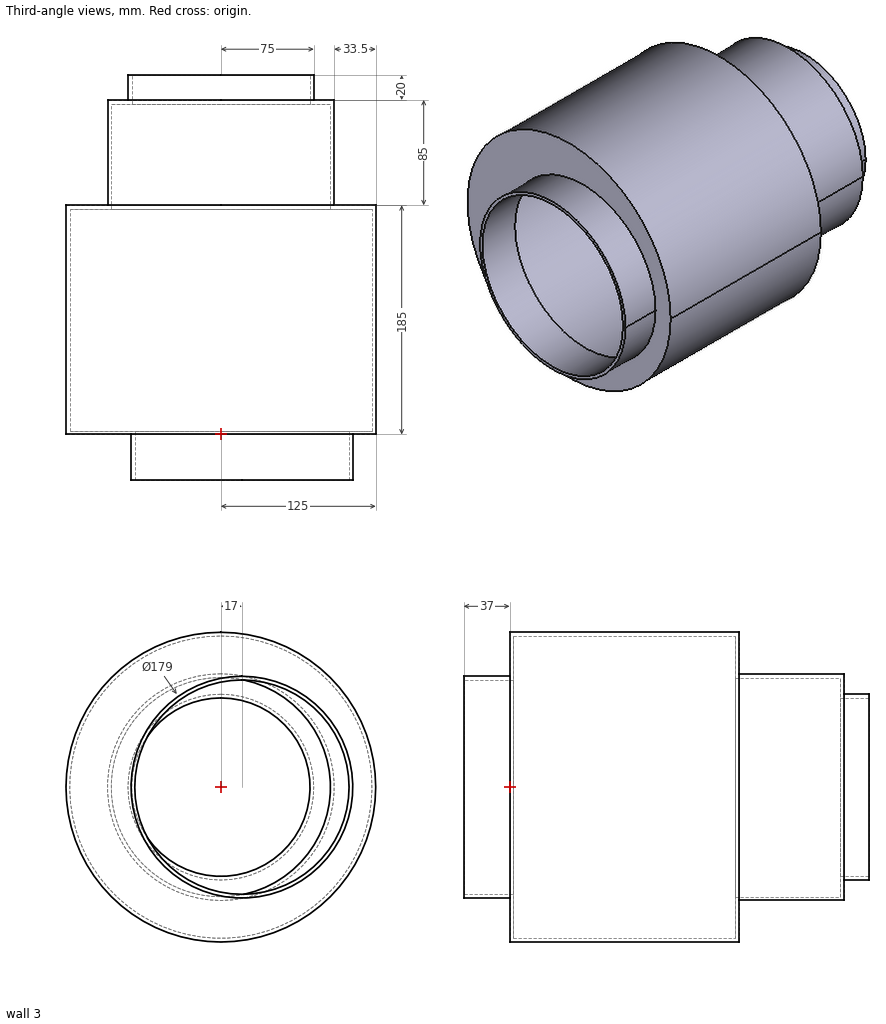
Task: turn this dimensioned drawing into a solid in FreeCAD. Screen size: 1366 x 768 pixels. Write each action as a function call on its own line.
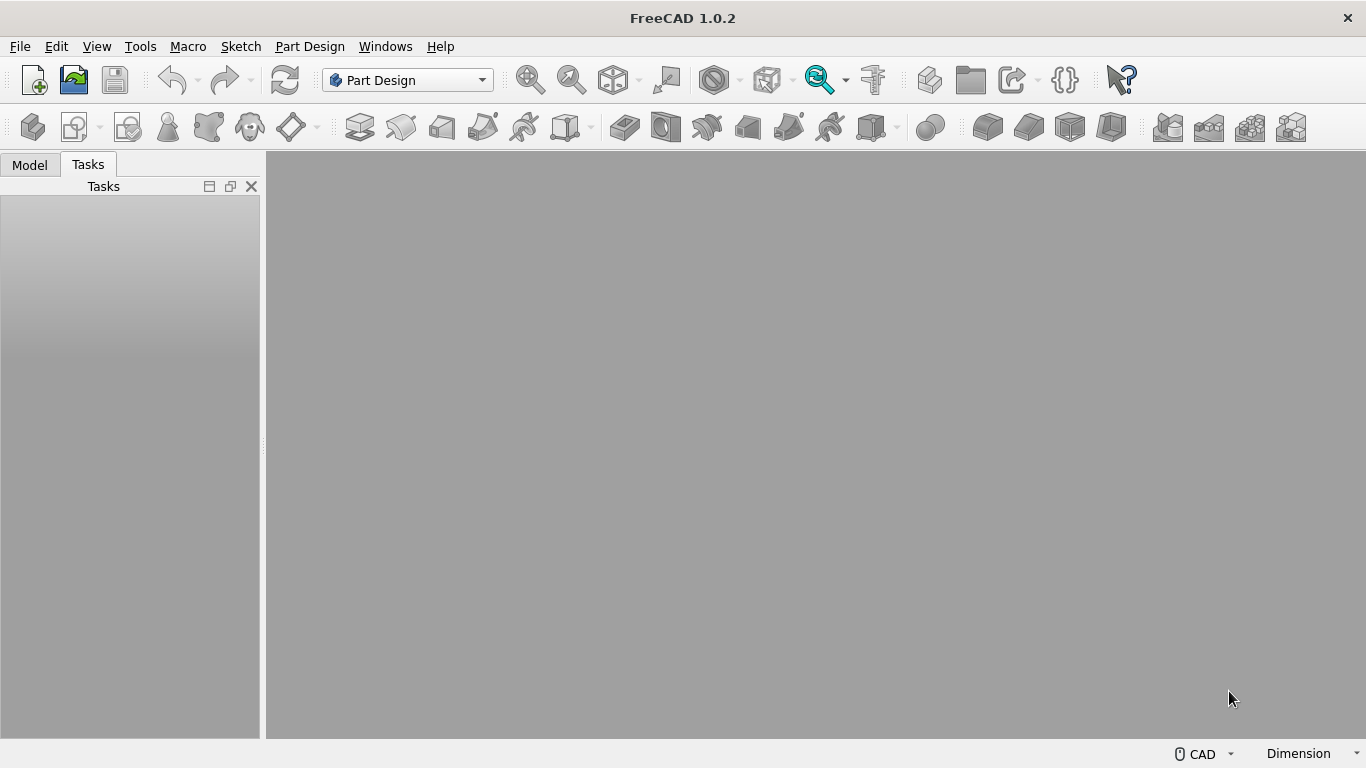
click(33, 80)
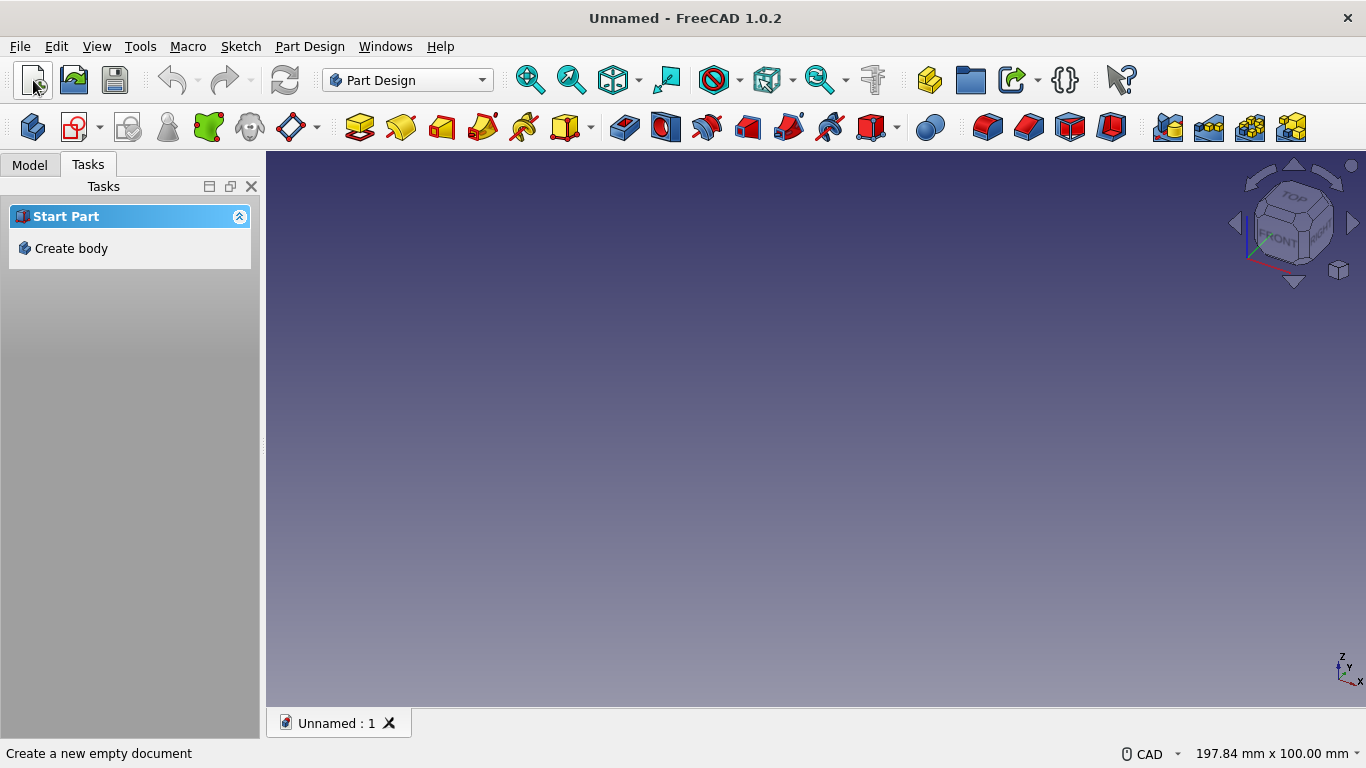
click(74, 128)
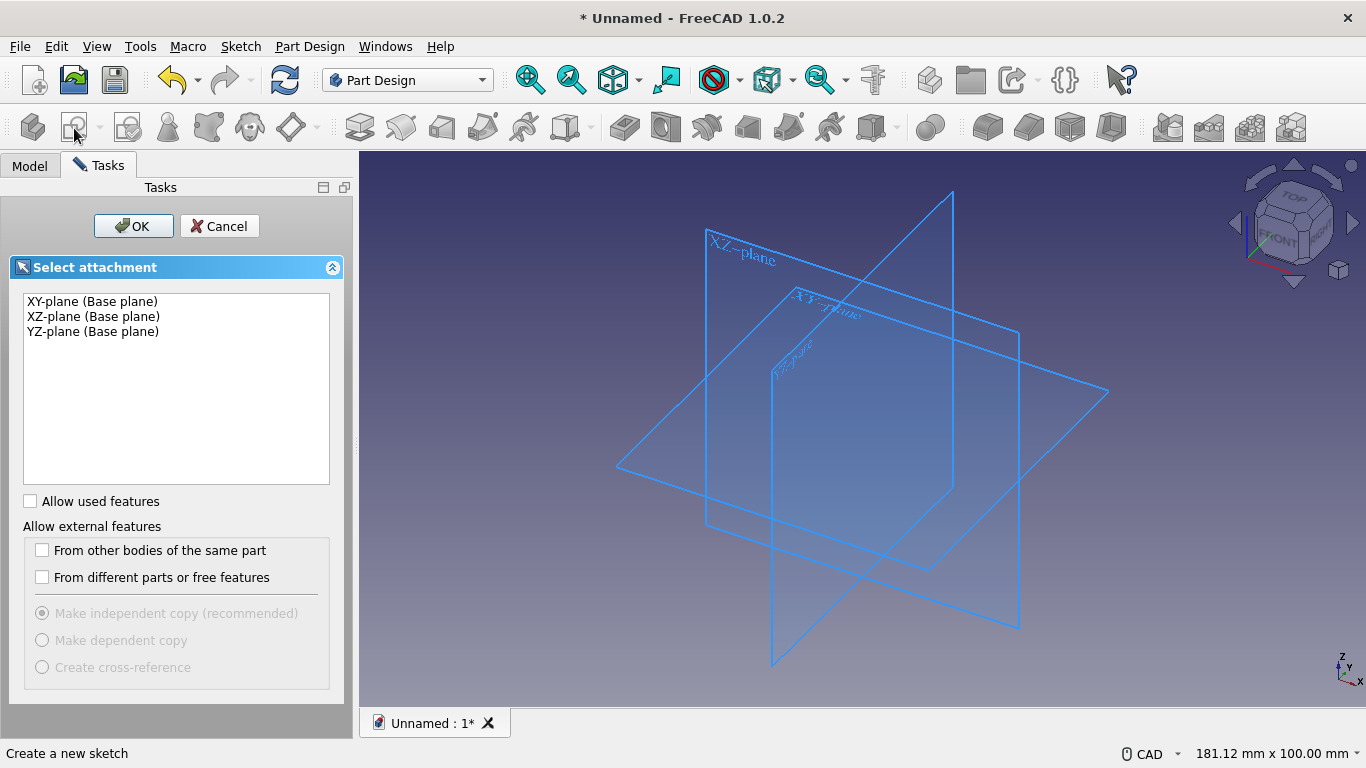
click(84, 302)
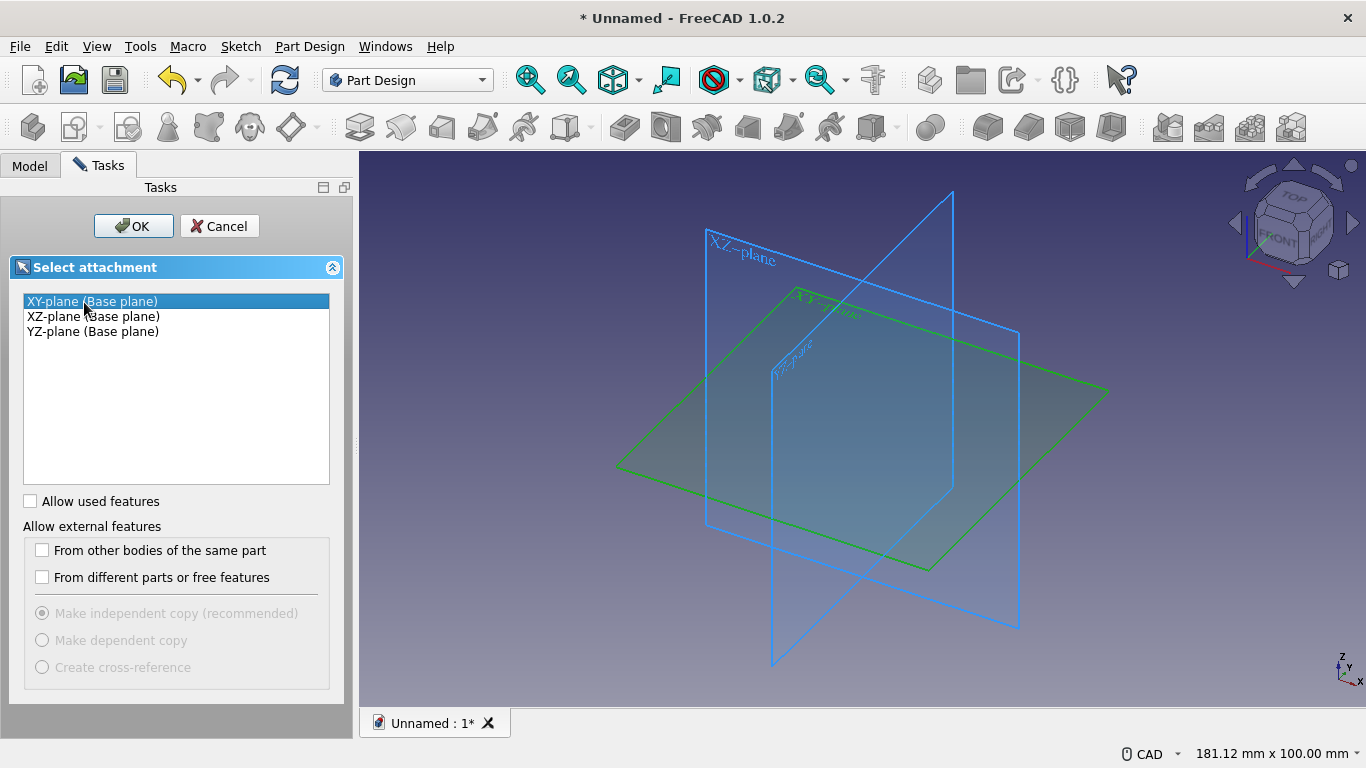
click(134, 226)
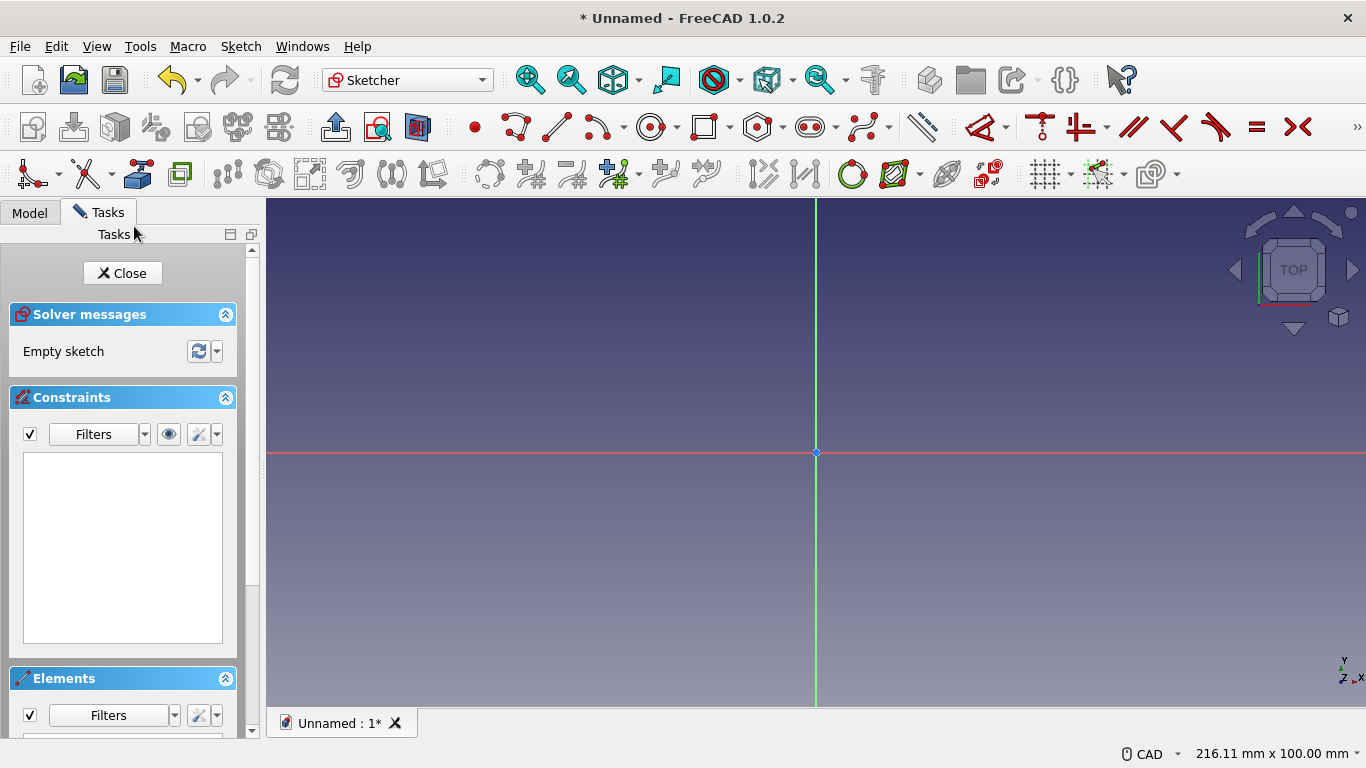
scroll(650, 639, down, 8)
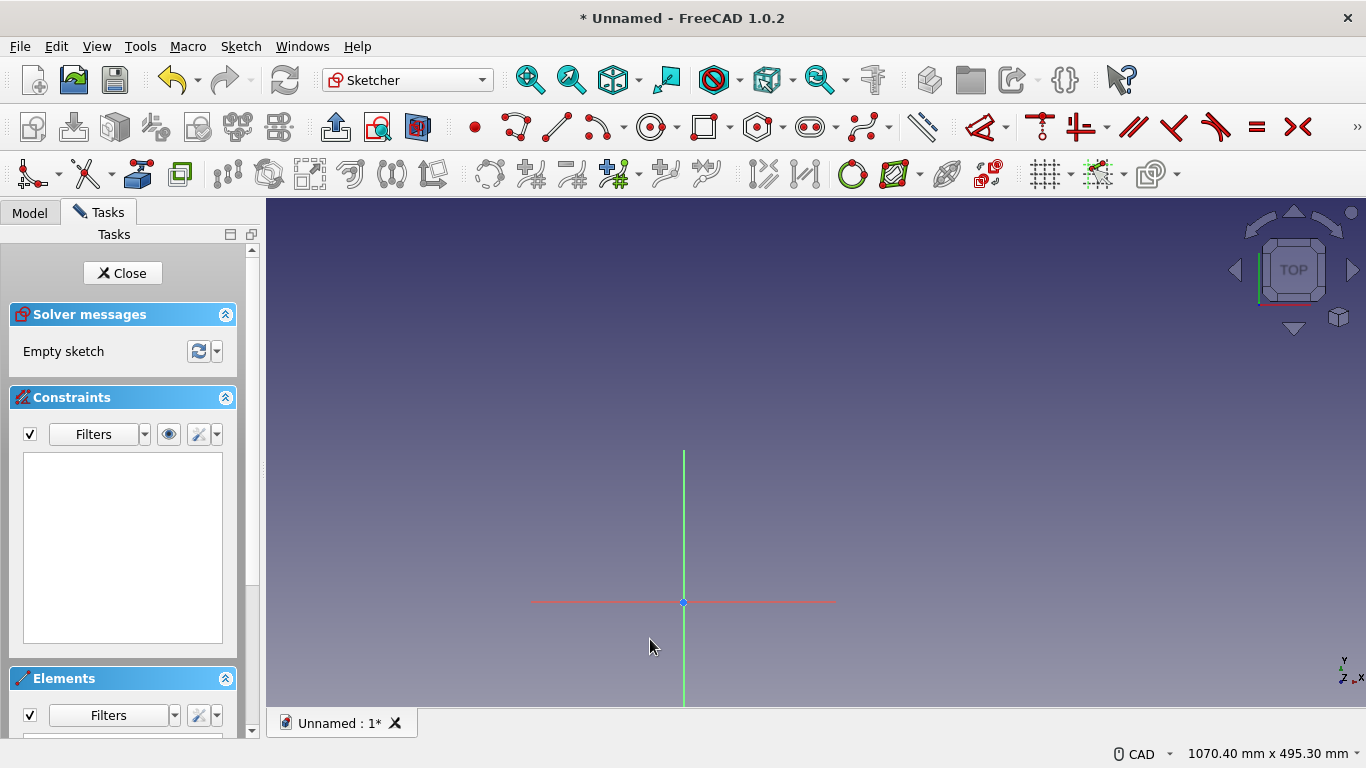
click(516, 128)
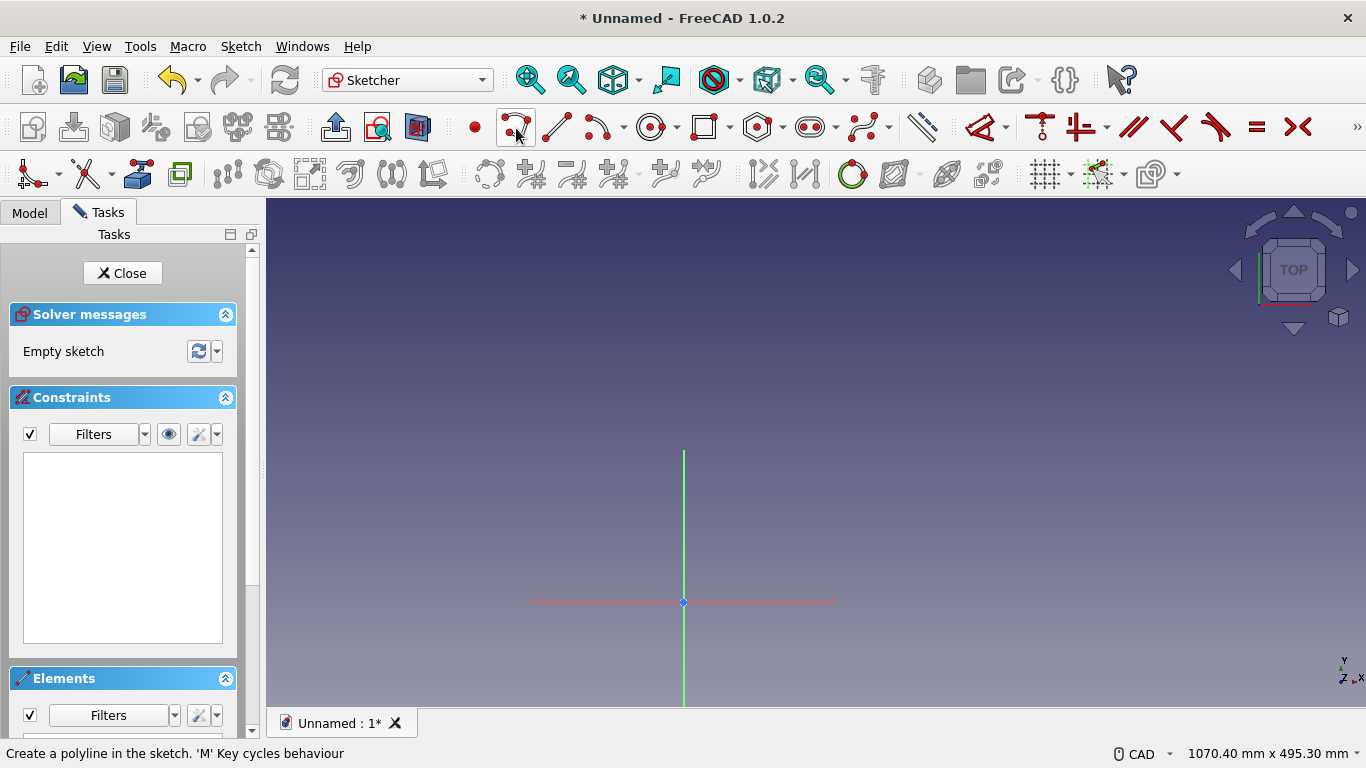
click(684, 602)
click(812, 593)
click(812, 412)
click(778, 412)
click(778, 325)
click(761, 325)
click(761, 304)
click(693, 304)
click(684, 602)
key(Escape)
key(Escape)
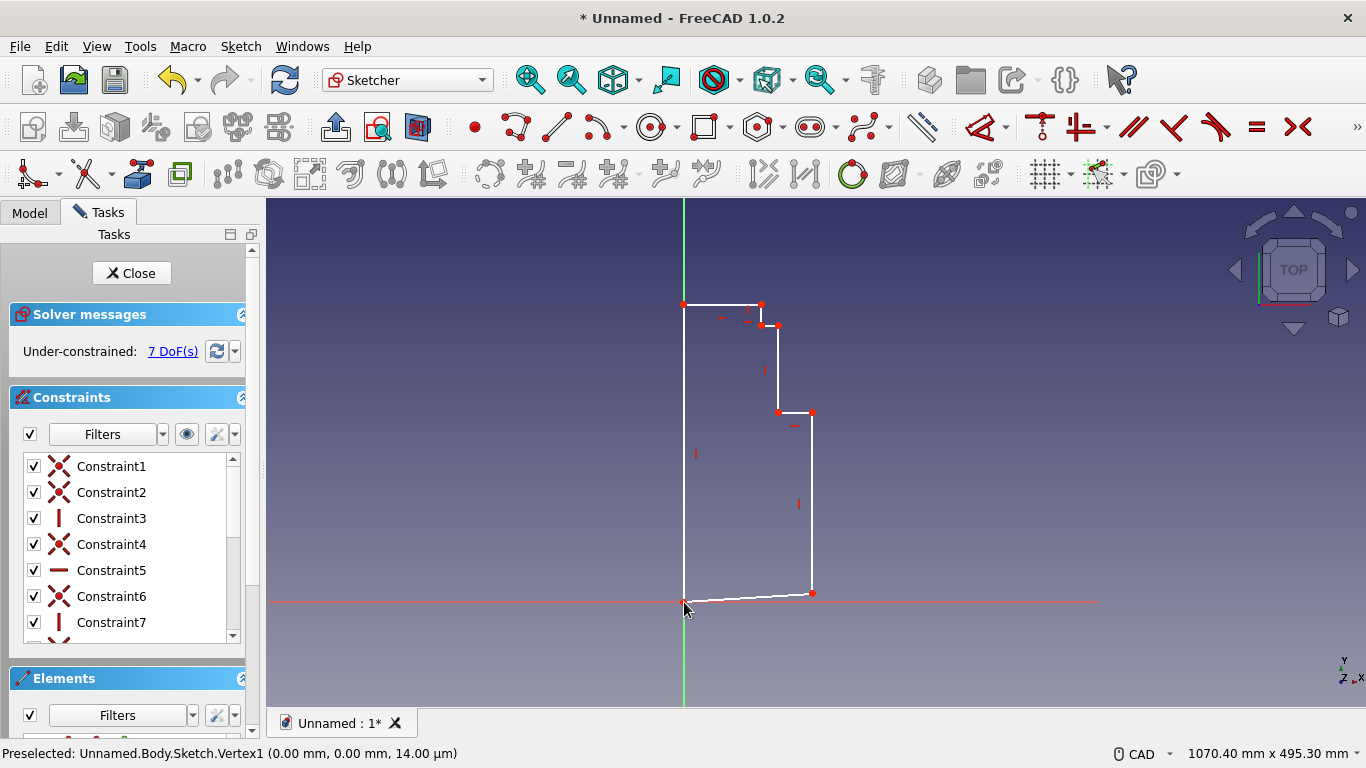
click(722, 600)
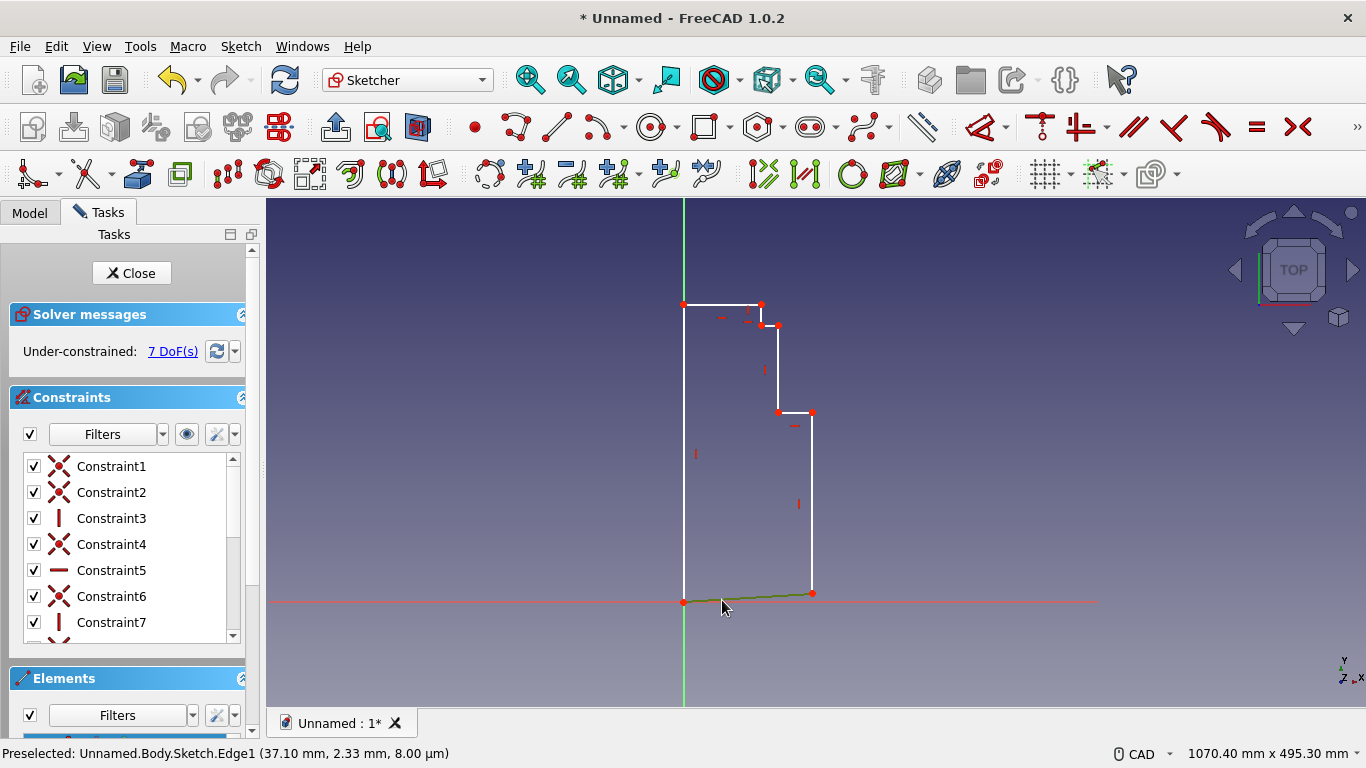
click(1106, 128)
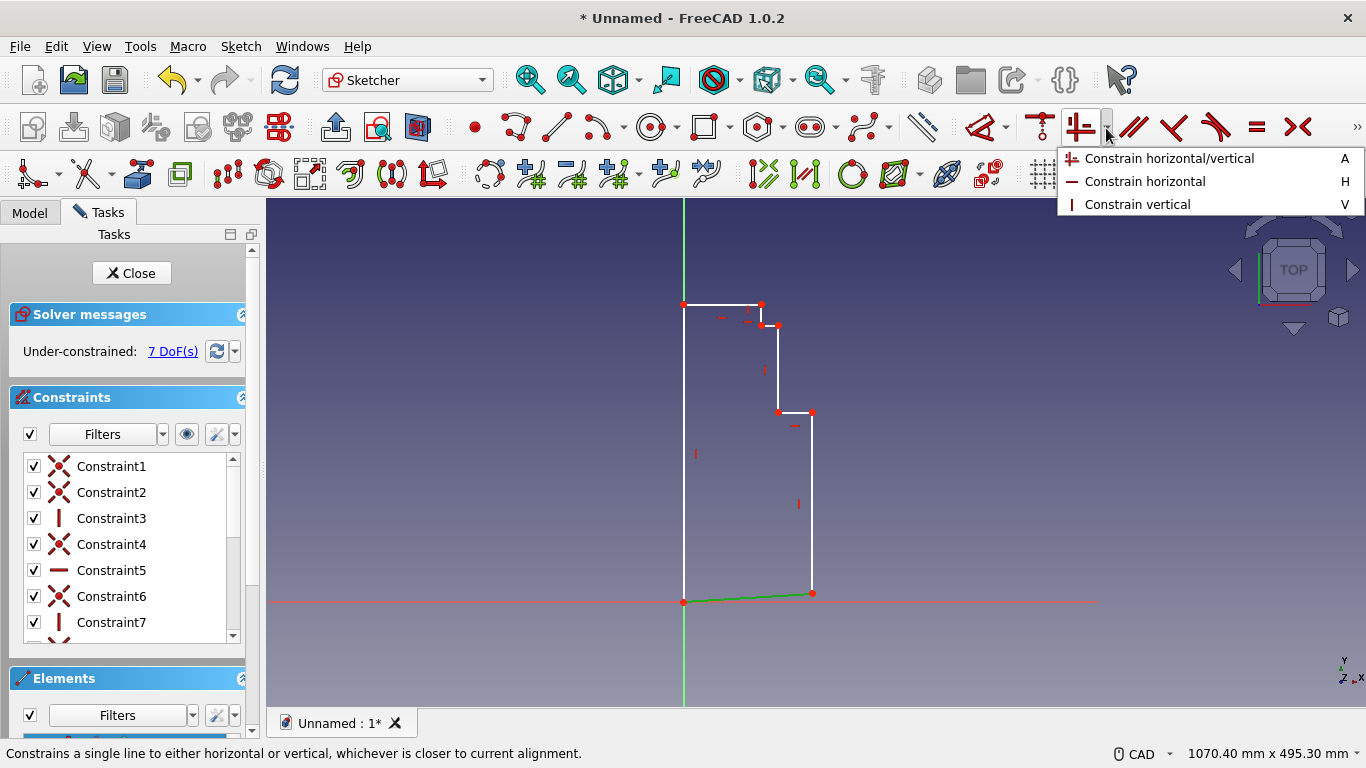
click(1211, 182)